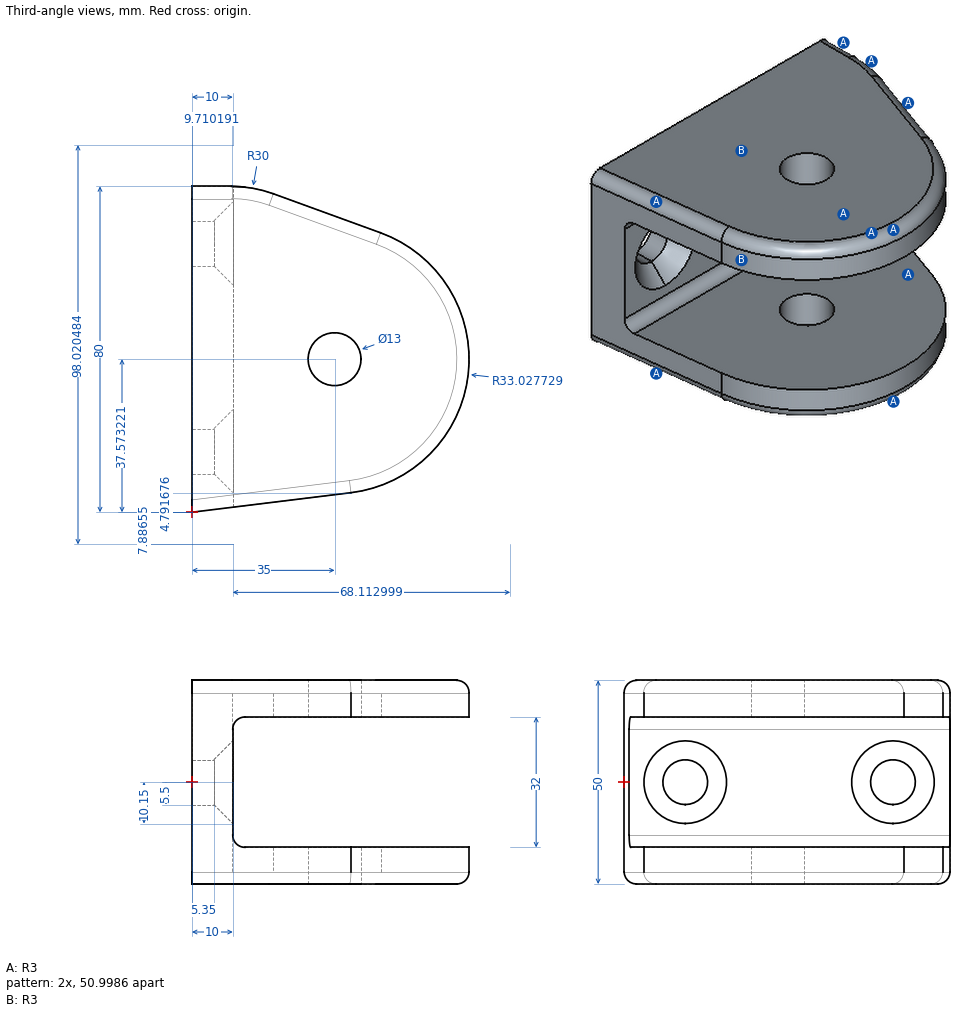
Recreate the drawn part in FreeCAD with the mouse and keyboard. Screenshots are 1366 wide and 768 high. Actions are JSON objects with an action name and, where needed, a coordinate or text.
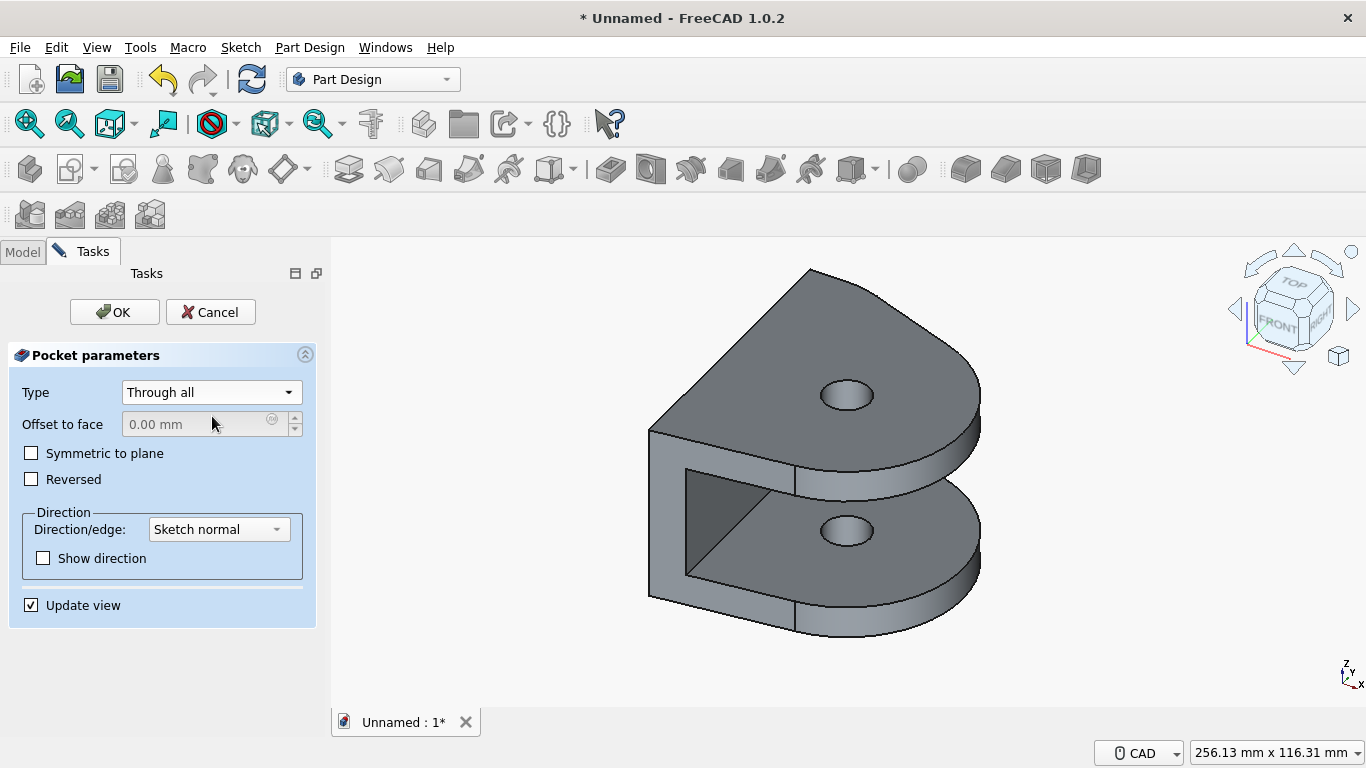
{"action": "left_click", "coordinate": [115, 312]}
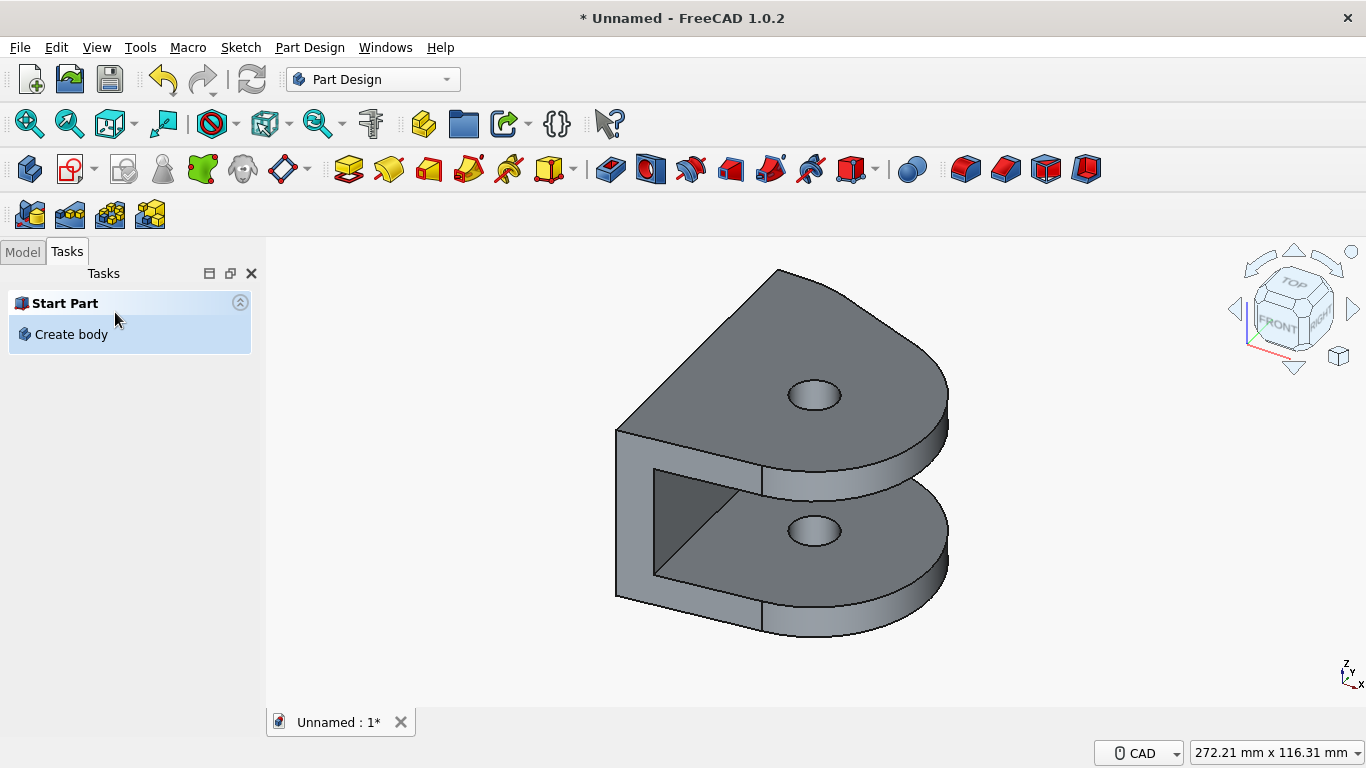
{"action": "left_click", "coordinate": [832, 288]}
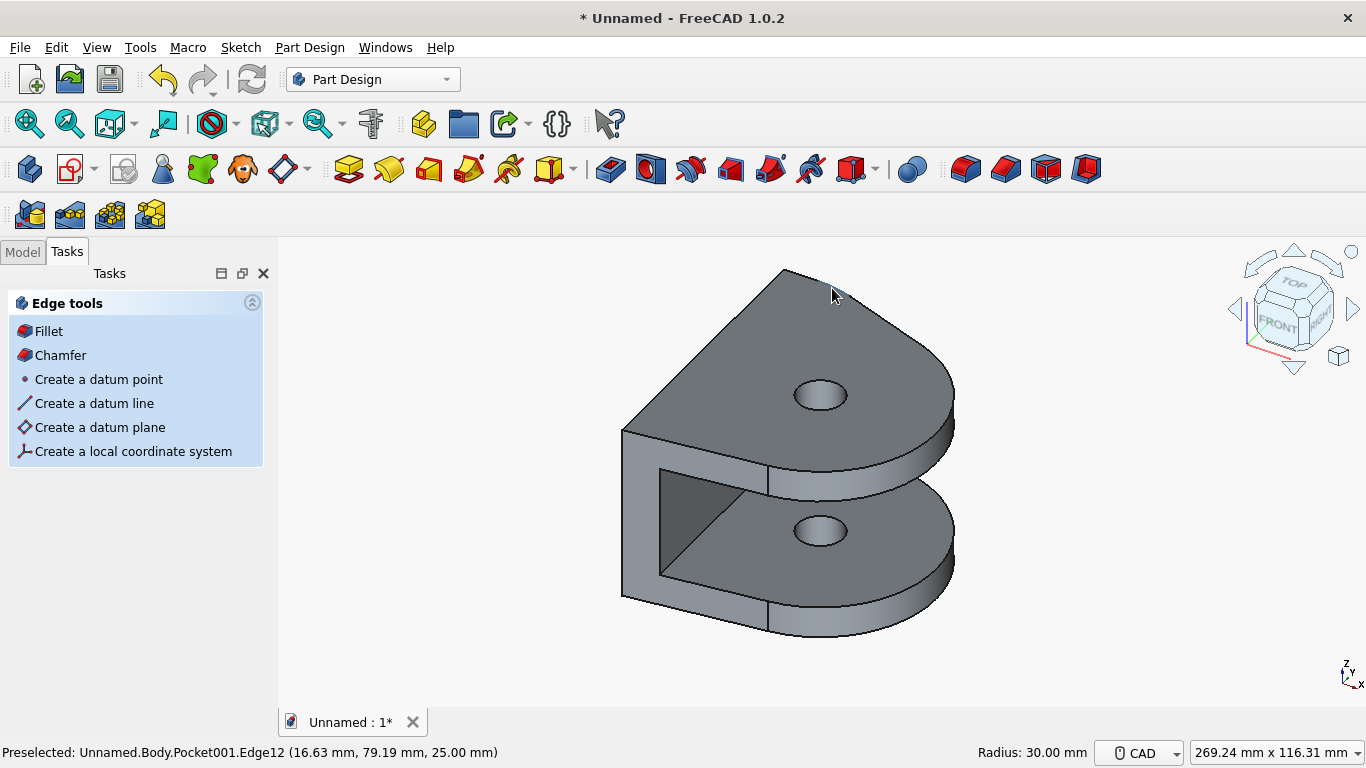
{"action": "left_click", "coordinate": [695, 447], "text": "ctrl"}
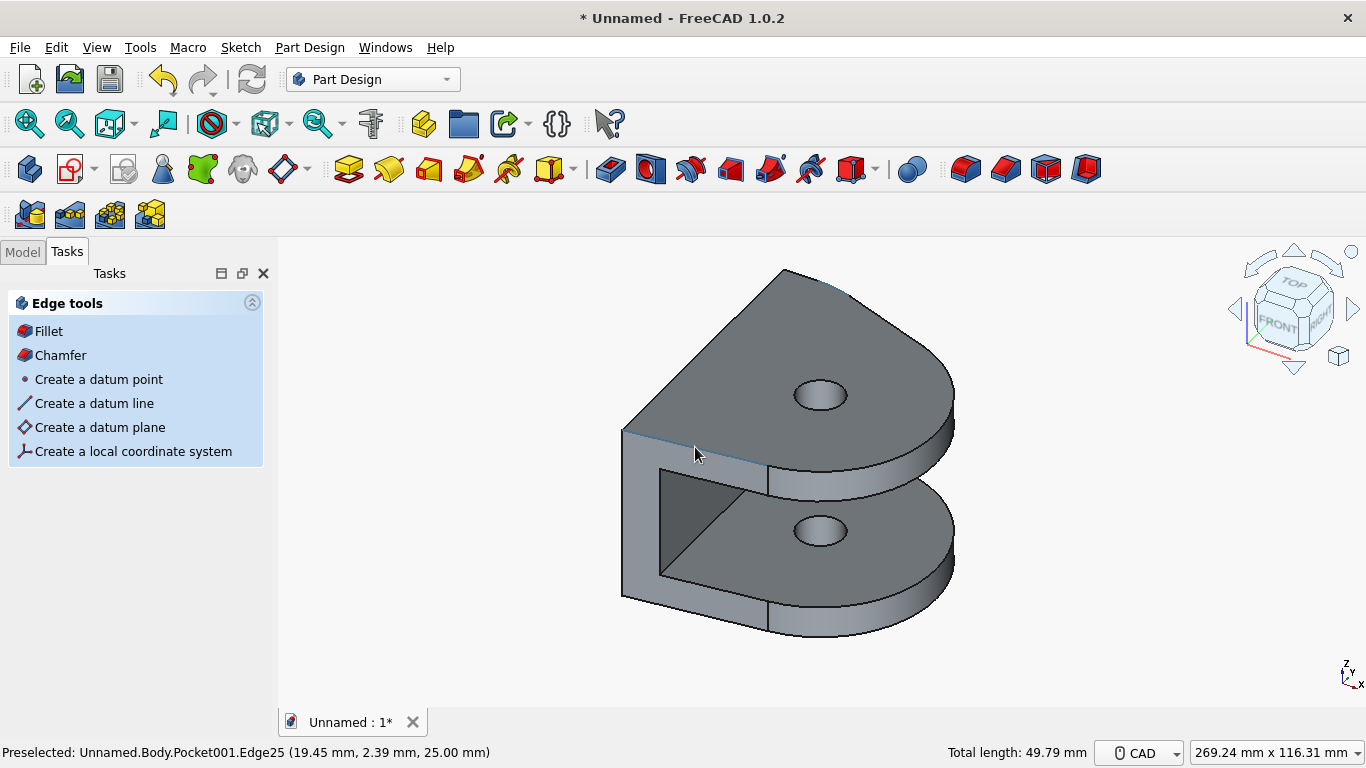
{"action": "left_click", "coordinate": [928, 440], "text": "ctrl"}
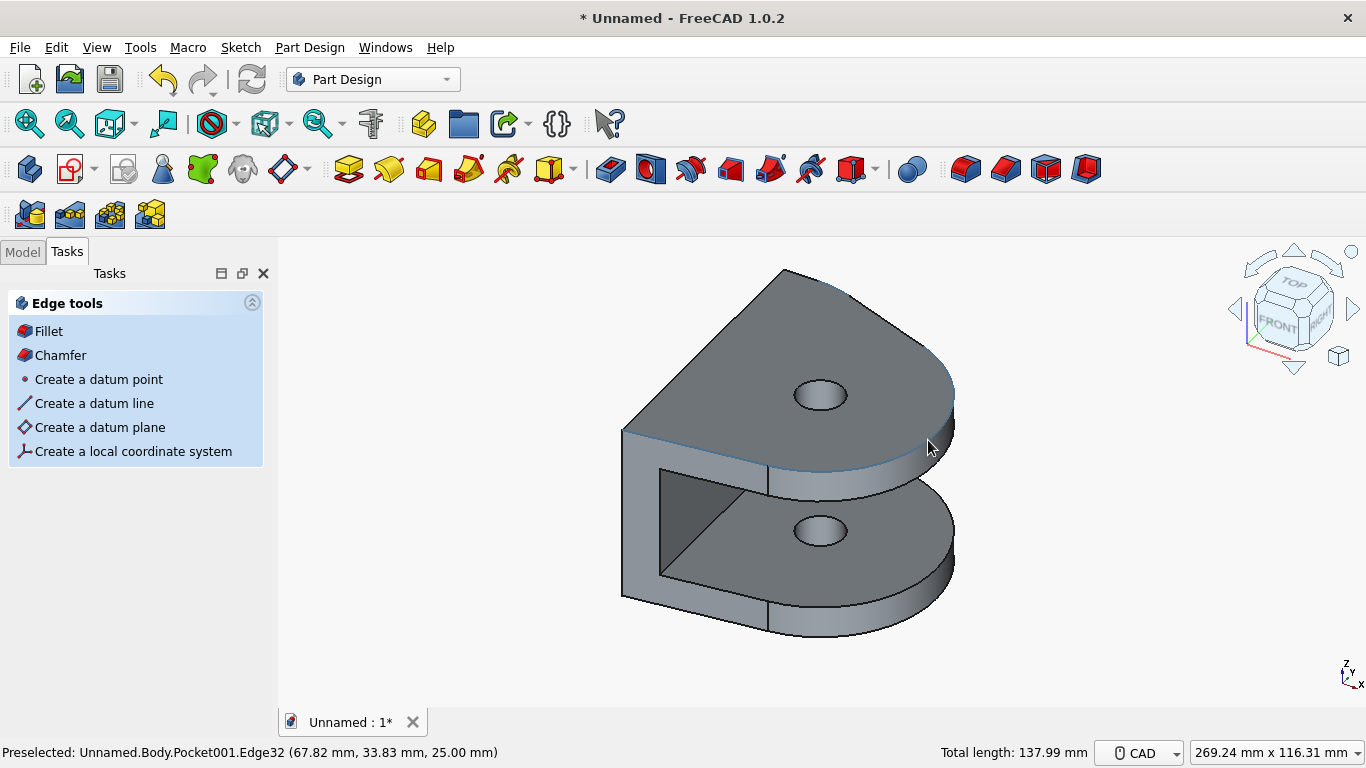
{"action": "key", "text": "0"}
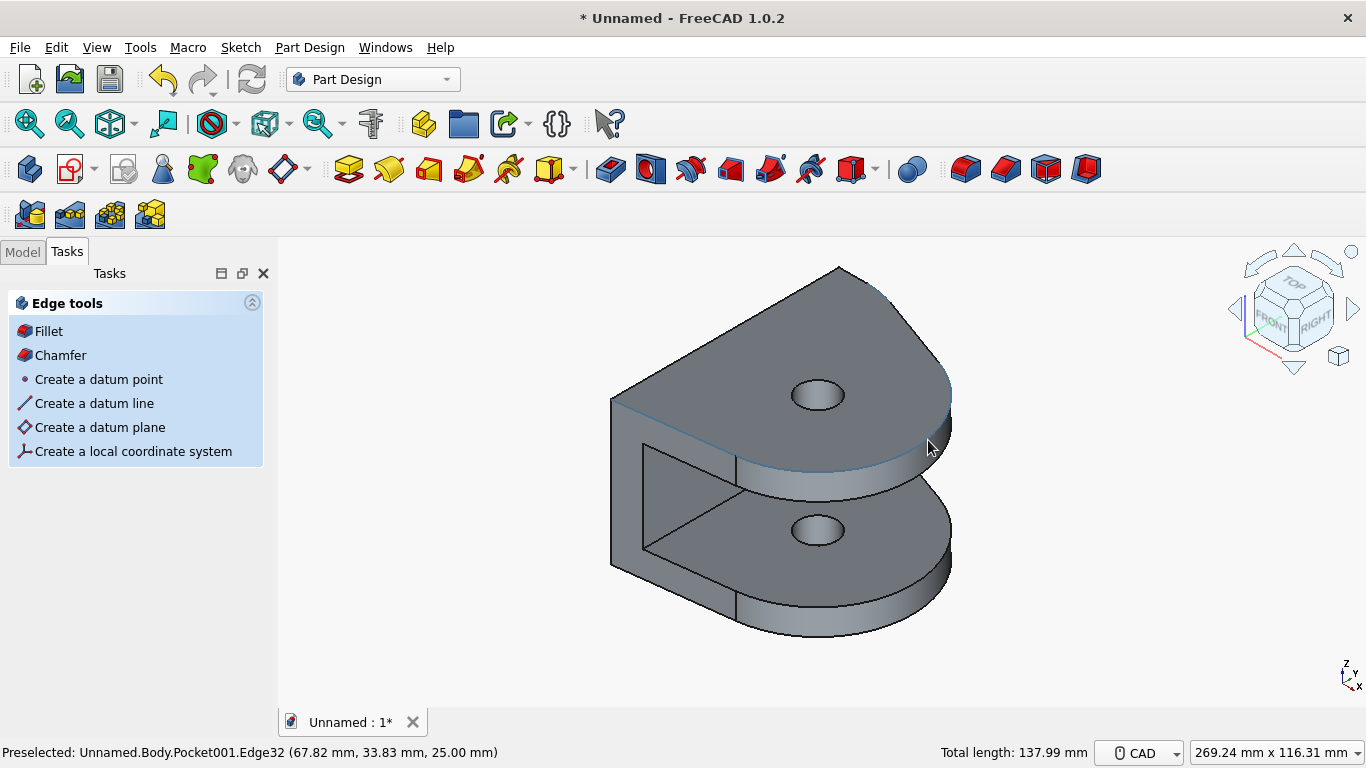
{"action": "left_click", "coordinate": [926, 605], "text": "ctrl"}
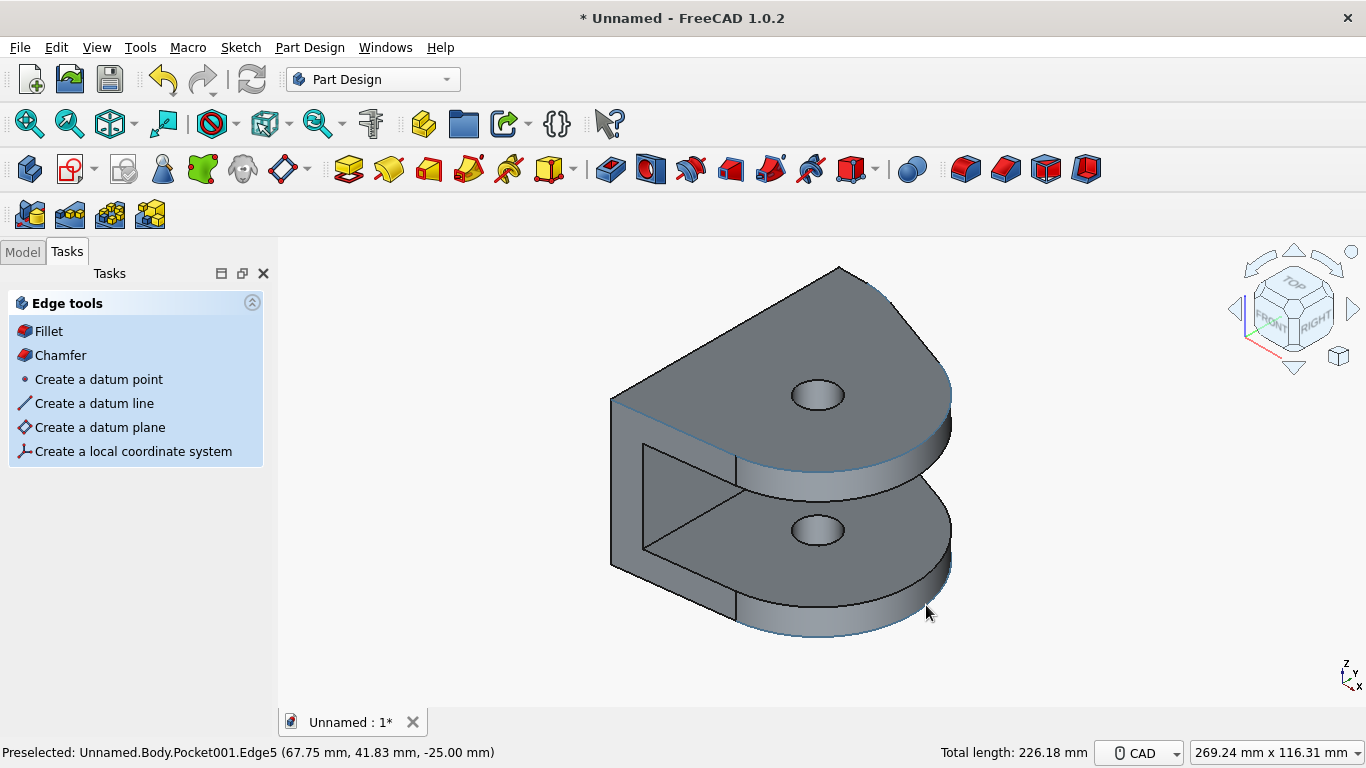
{"action": "key", "text": "2"}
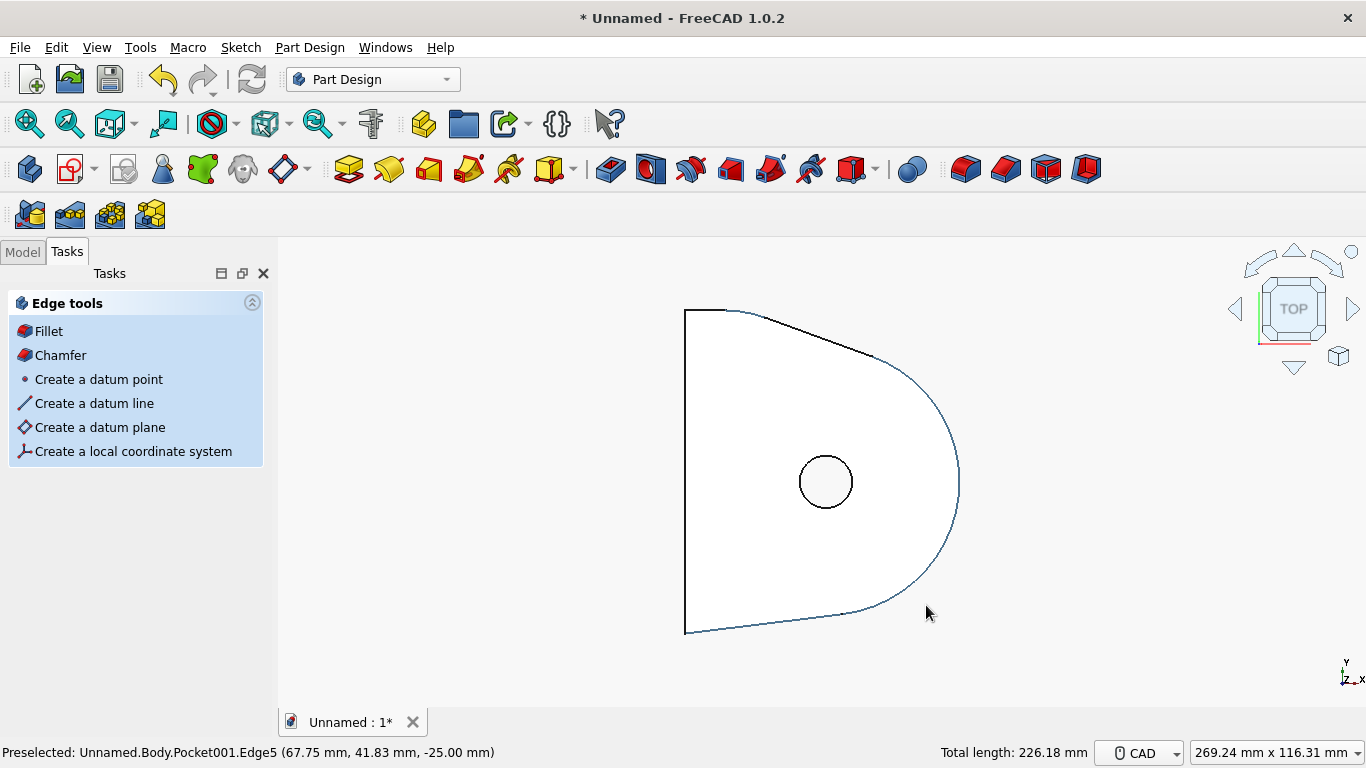
{"action": "left_click", "coordinate": [818, 336], "text": "ctrl"}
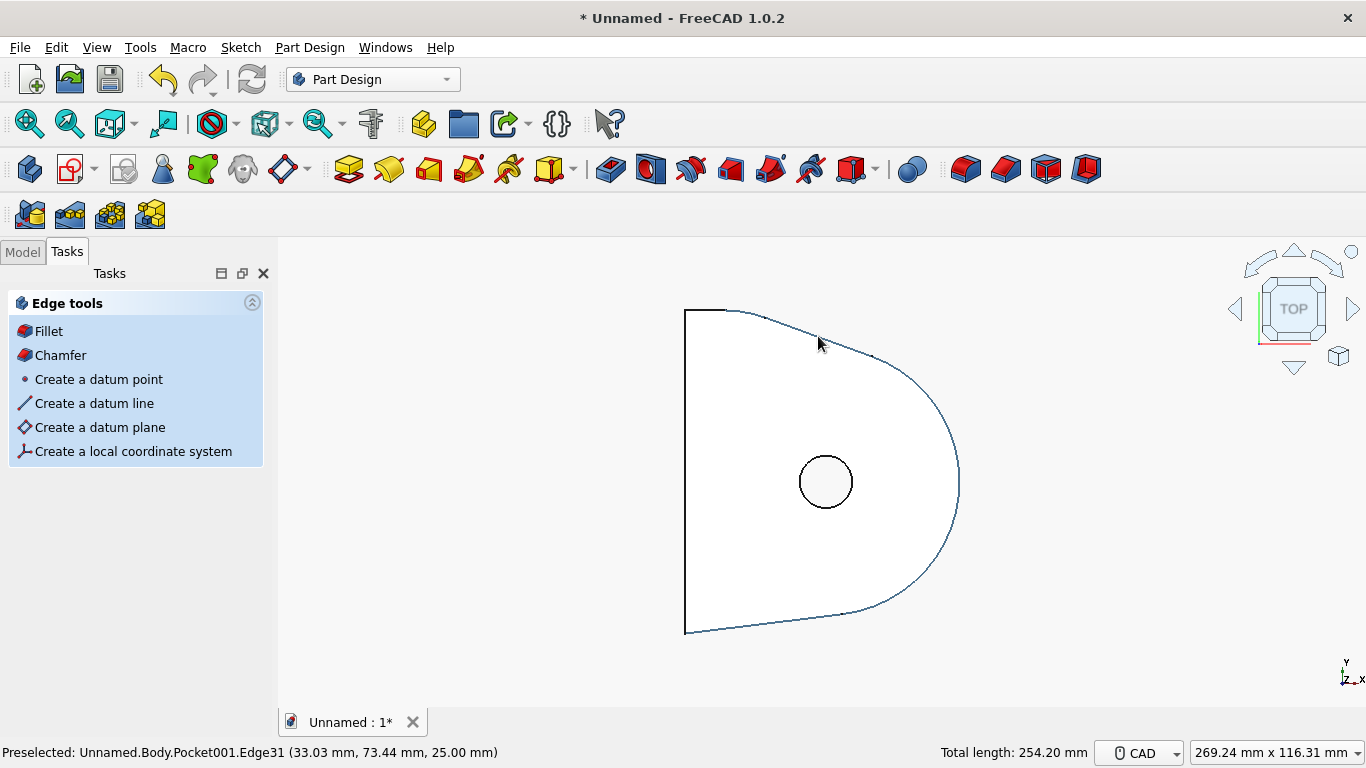
{"action": "left_click", "coordinate": [704, 309], "text": "ctrl"}